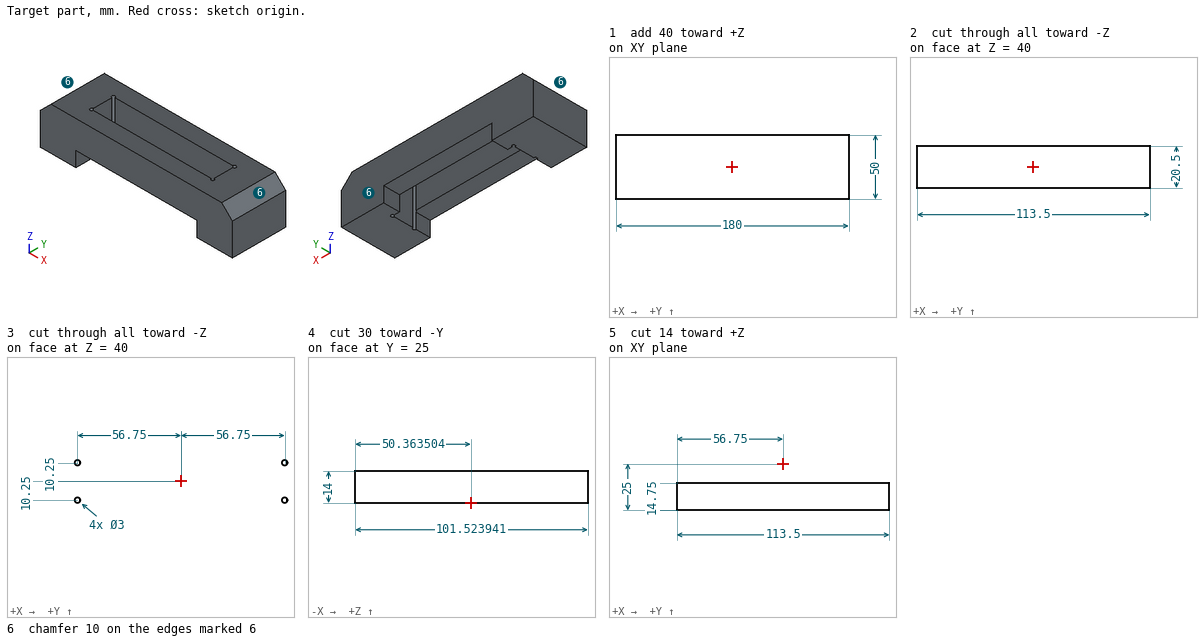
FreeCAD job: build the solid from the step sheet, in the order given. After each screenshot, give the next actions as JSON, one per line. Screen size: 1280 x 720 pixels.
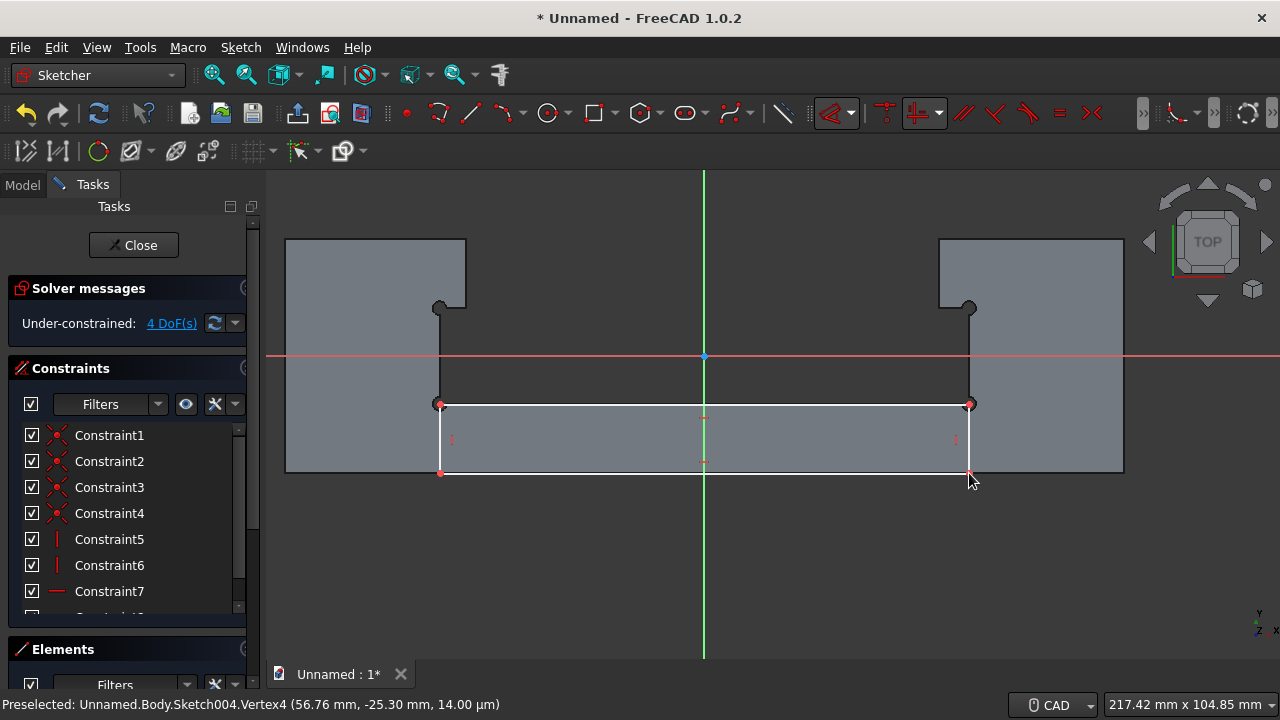
{"action": "left_click", "coordinate": [440, 474]}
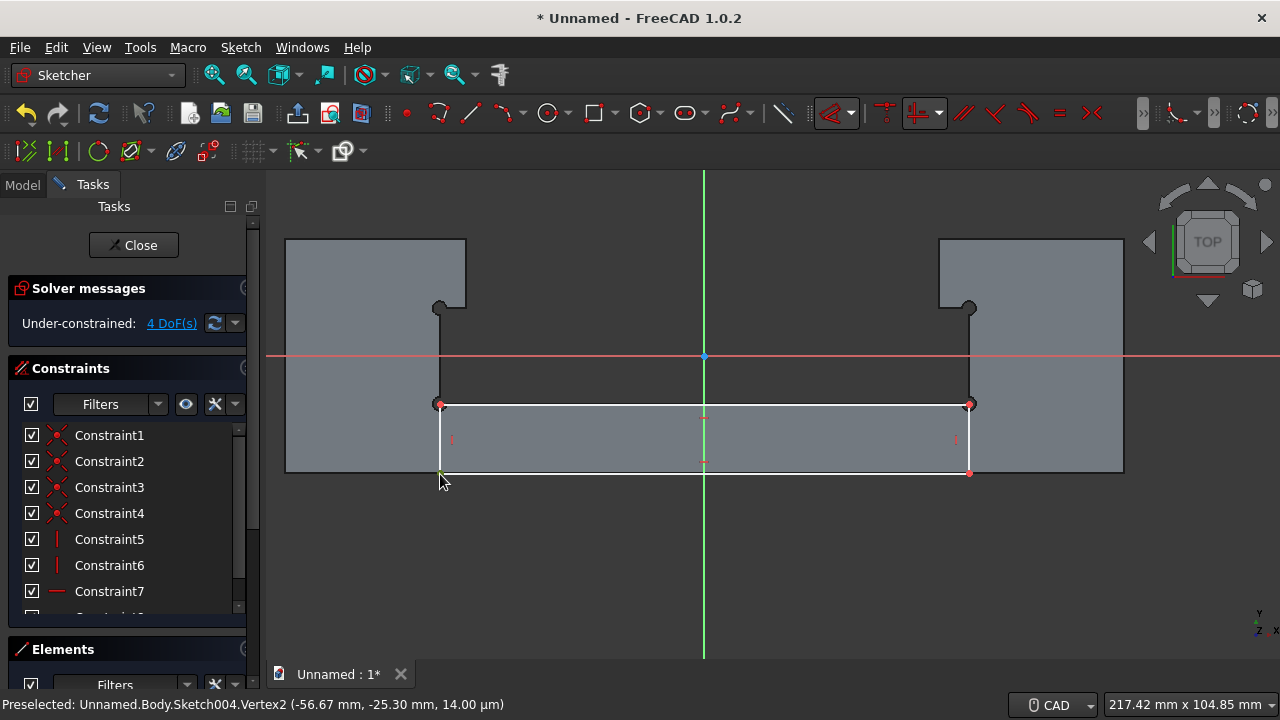
{"action": "left_click", "coordinate": [854, 114]}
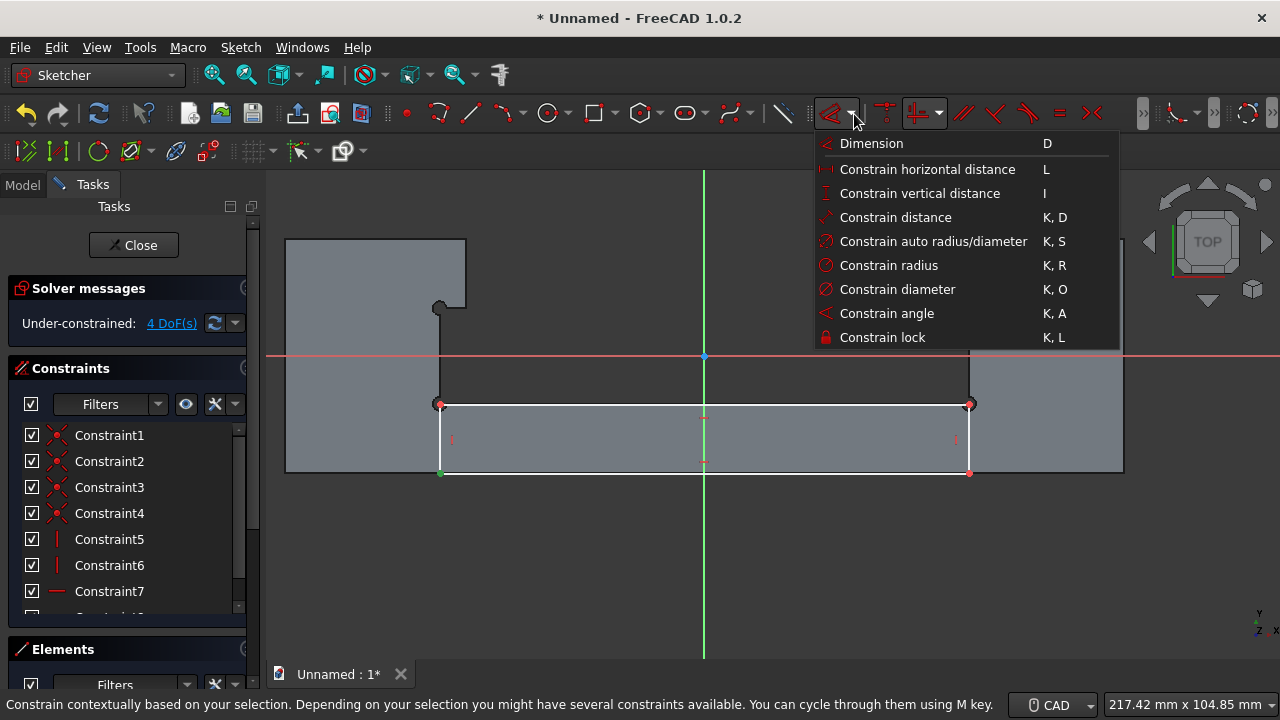
{"action": "left_click", "coordinate": [967, 193]}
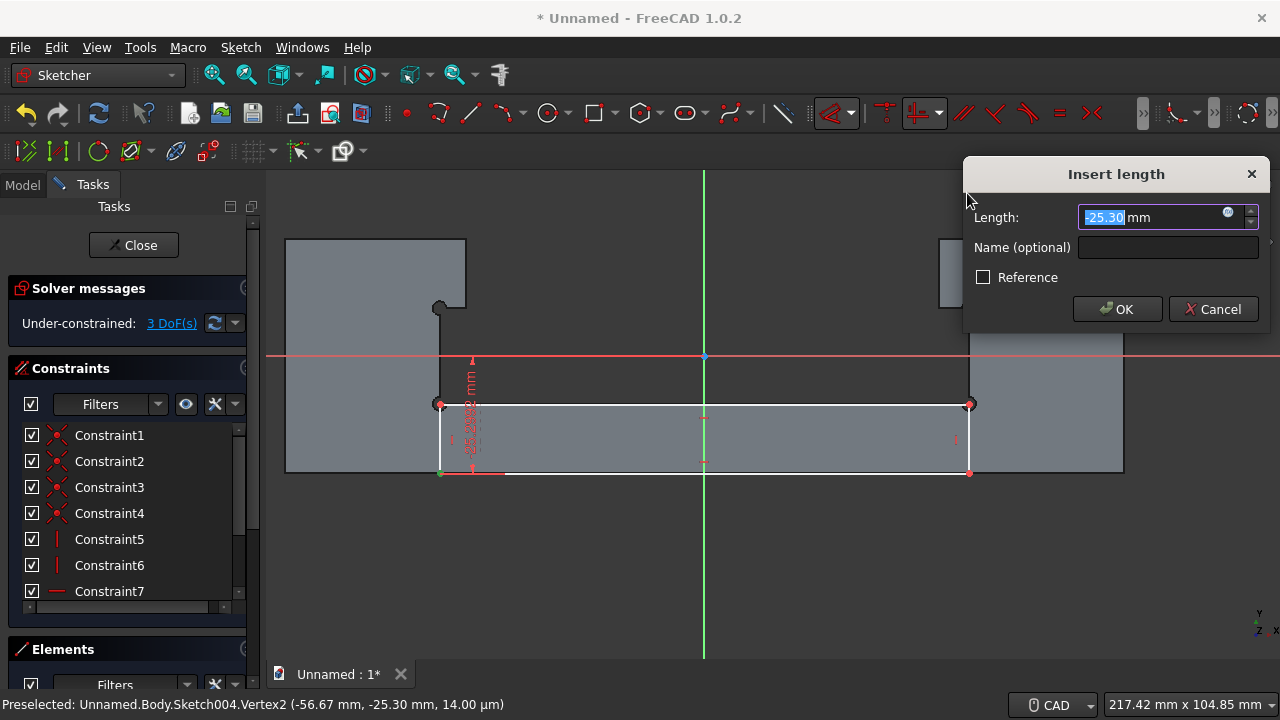
{"action": "type", "text": "-25"}
{"action": "key", "text": "Return"}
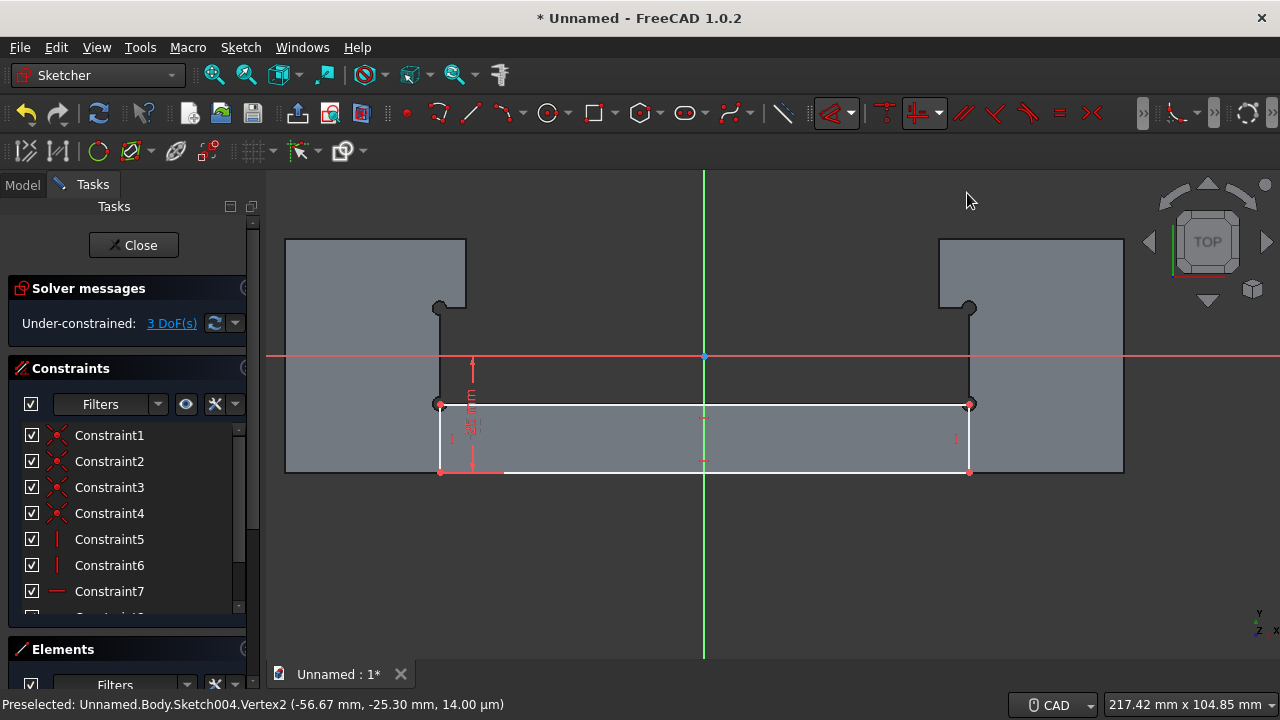
{"action": "left_click", "coordinate": [440, 425]}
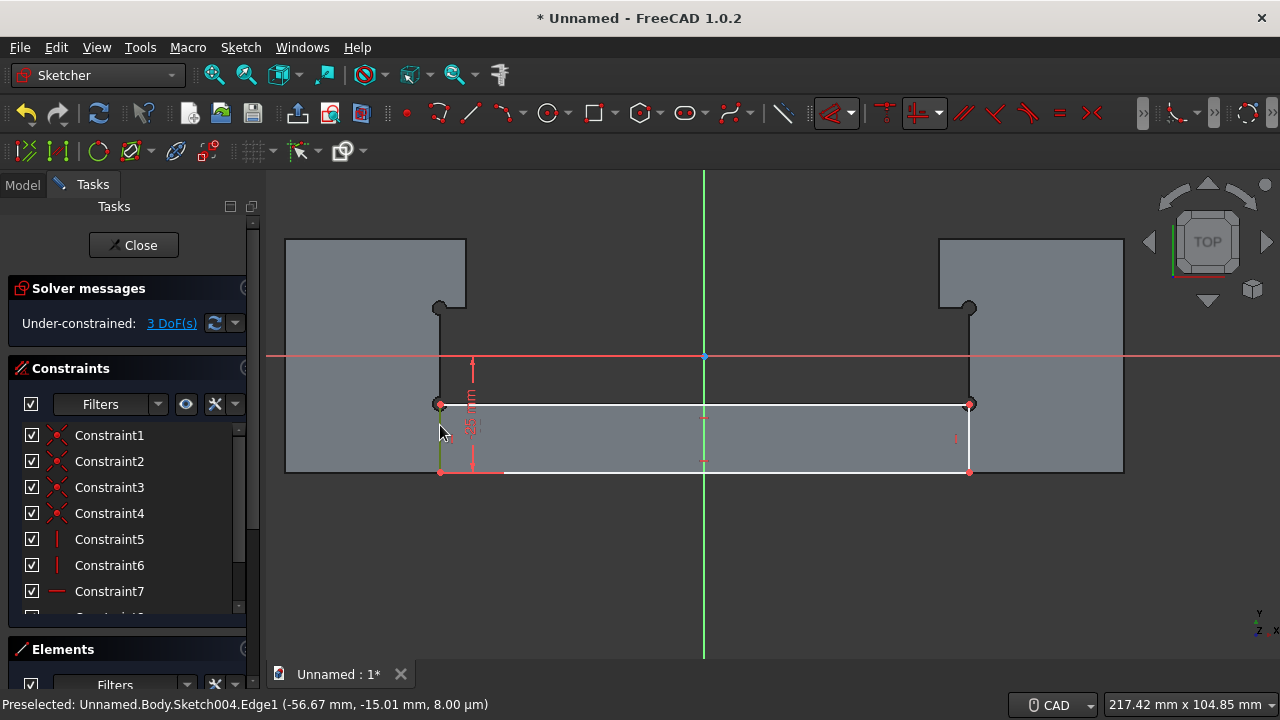
{"action": "key", "text": "i"}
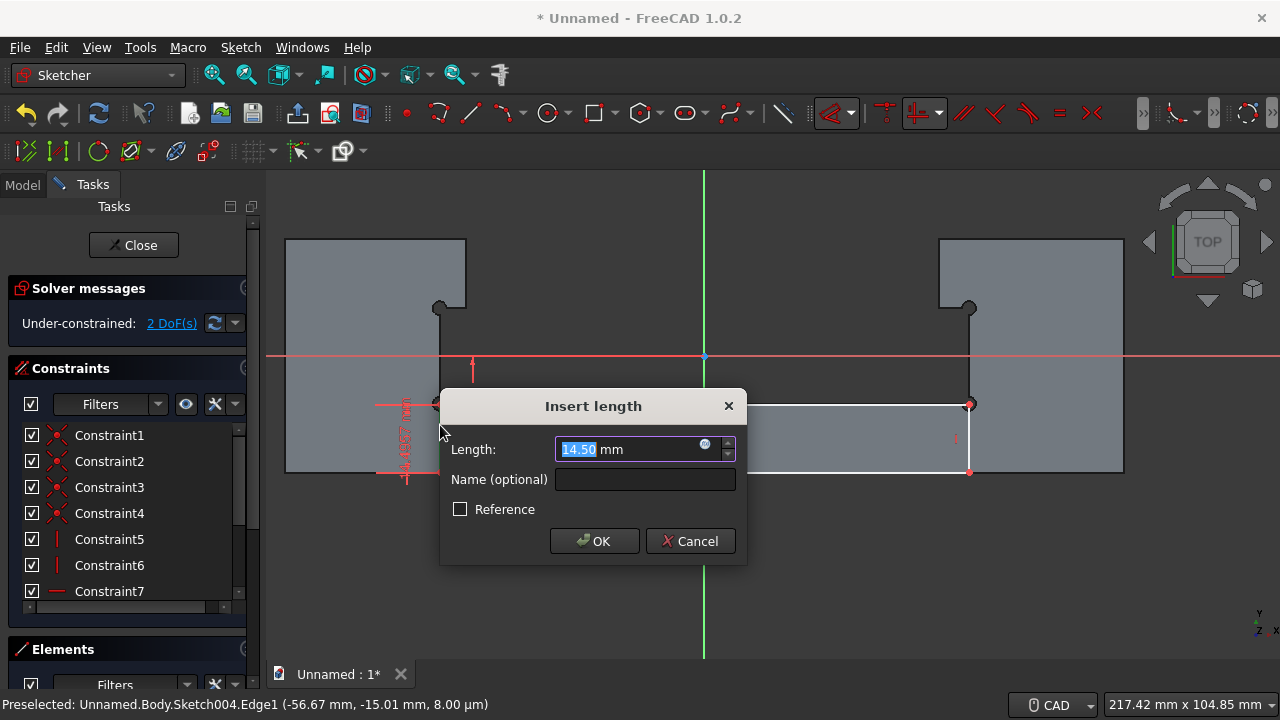
{"action": "type", "text": "14.75"}
{"action": "key", "text": "Return"}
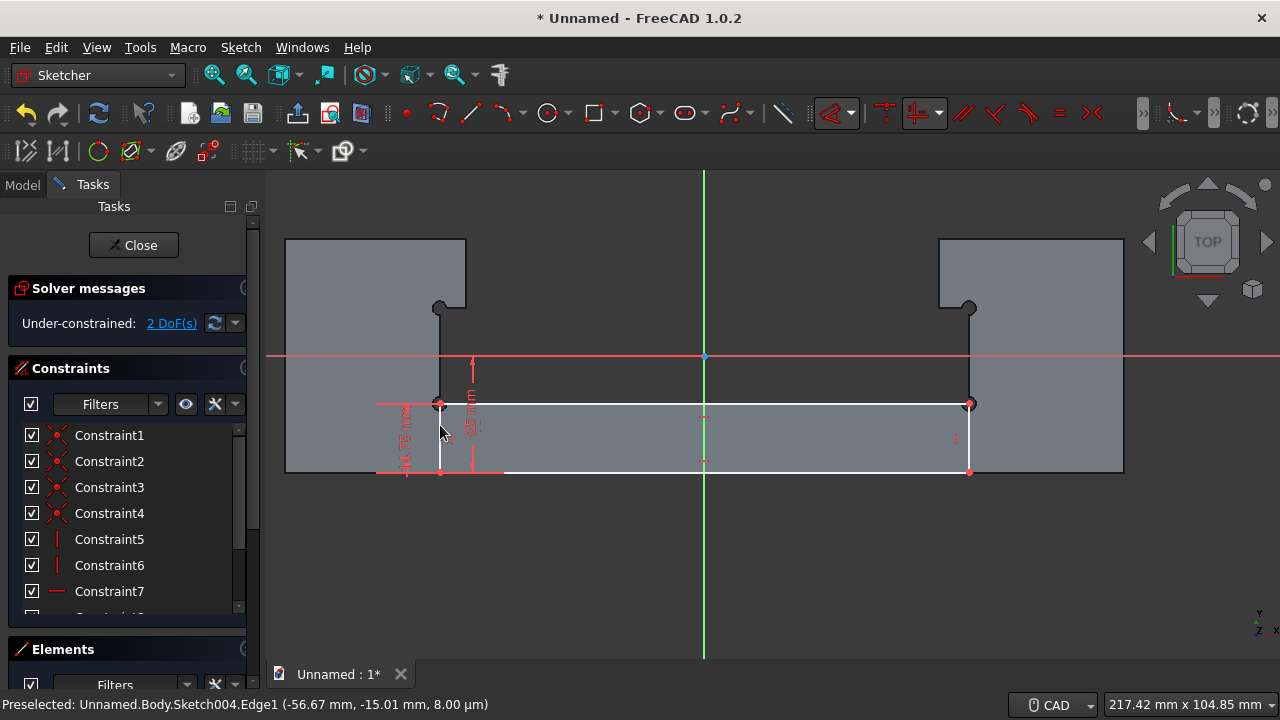
{"action": "left_click", "coordinate": [599, 473]}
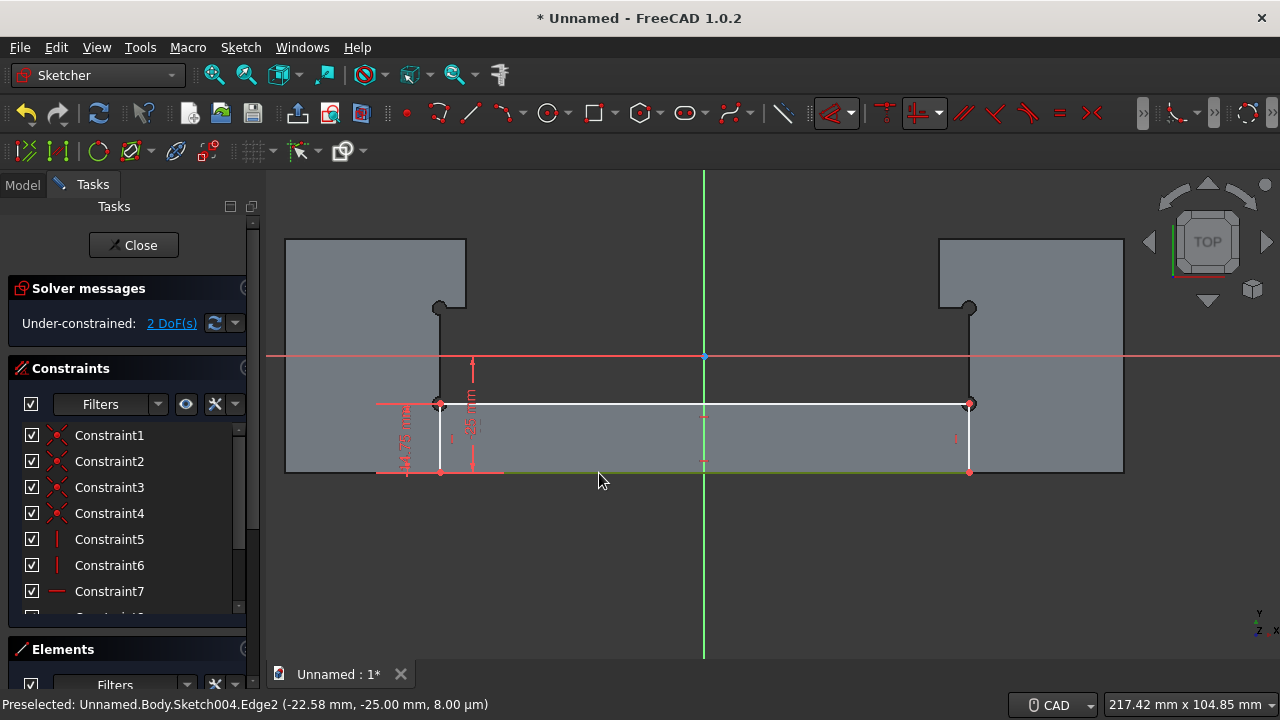
{"action": "key", "text": "l"}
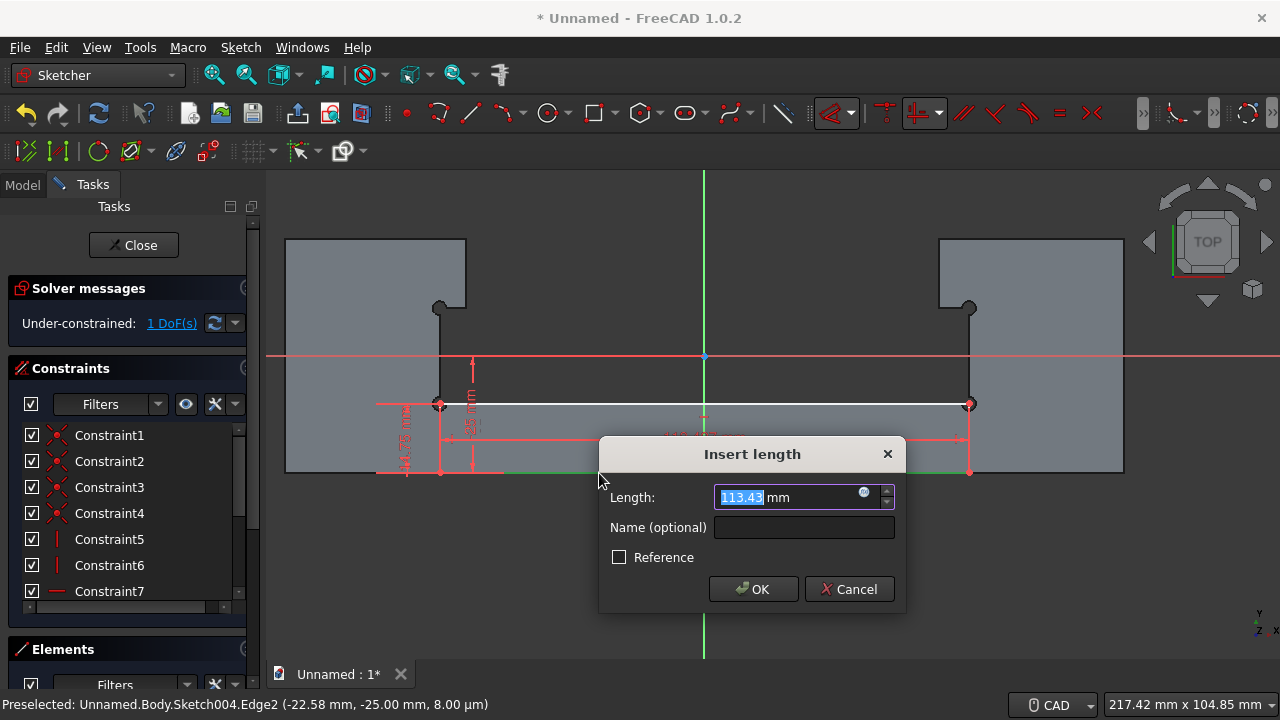
{"action": "type", "text": "113.5"}
{"action": "key", "text": "Return"}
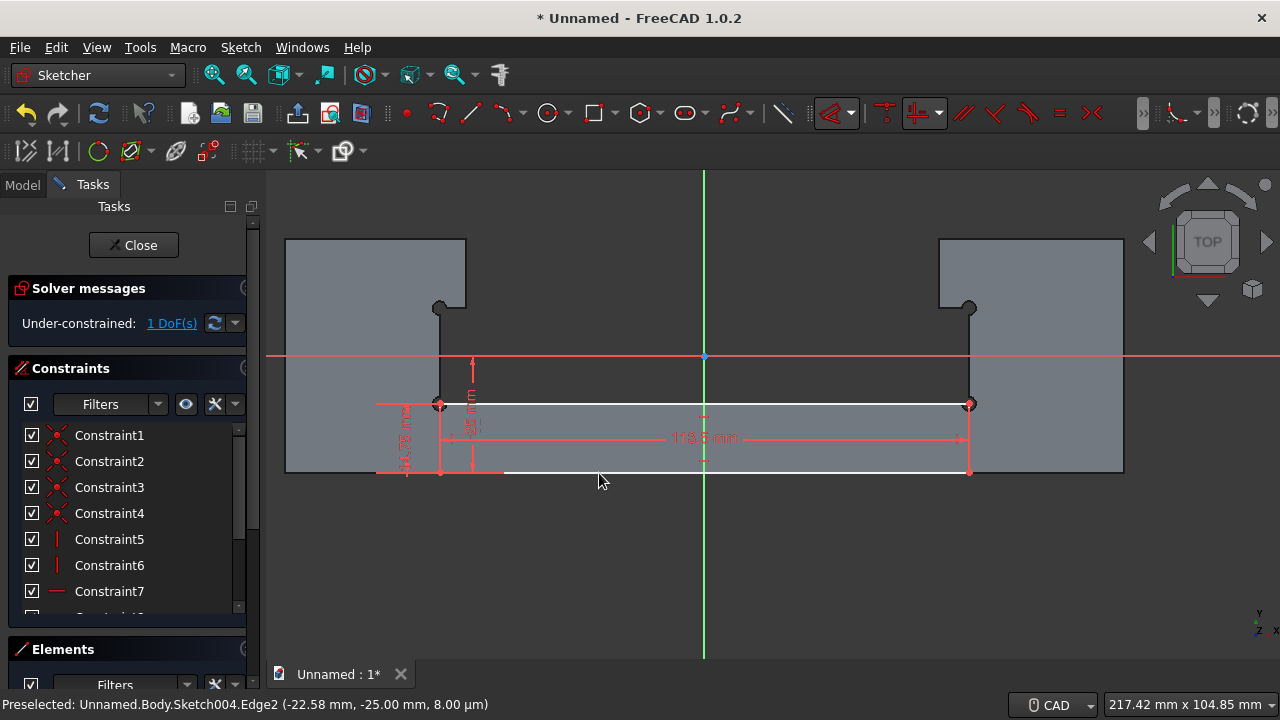
{"action": "left_click", "coordinate": [440, 404]}